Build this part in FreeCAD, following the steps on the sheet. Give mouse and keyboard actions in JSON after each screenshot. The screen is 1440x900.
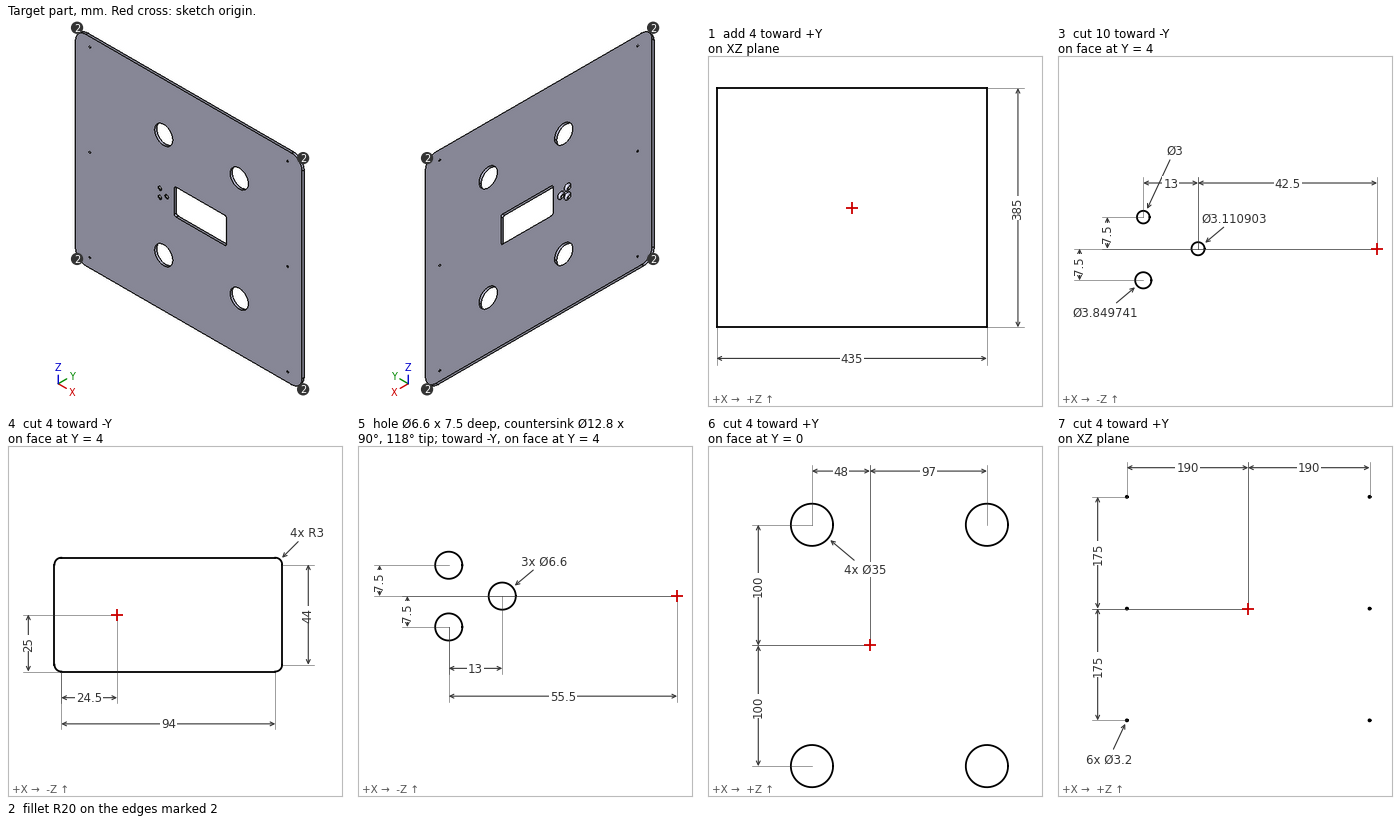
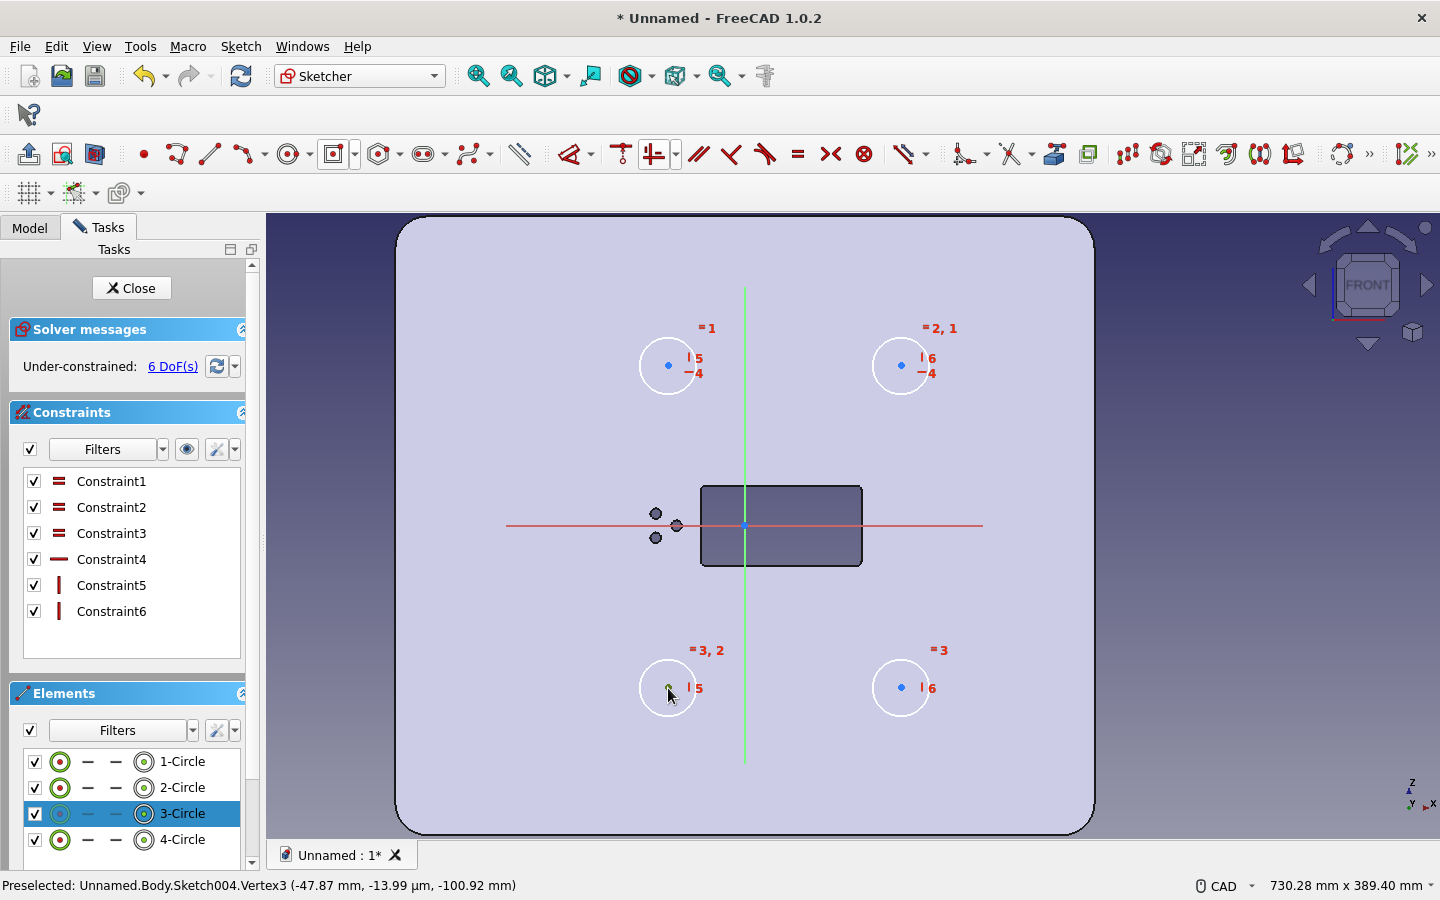
{"action": "left_click", "coordinate": [901, 688]}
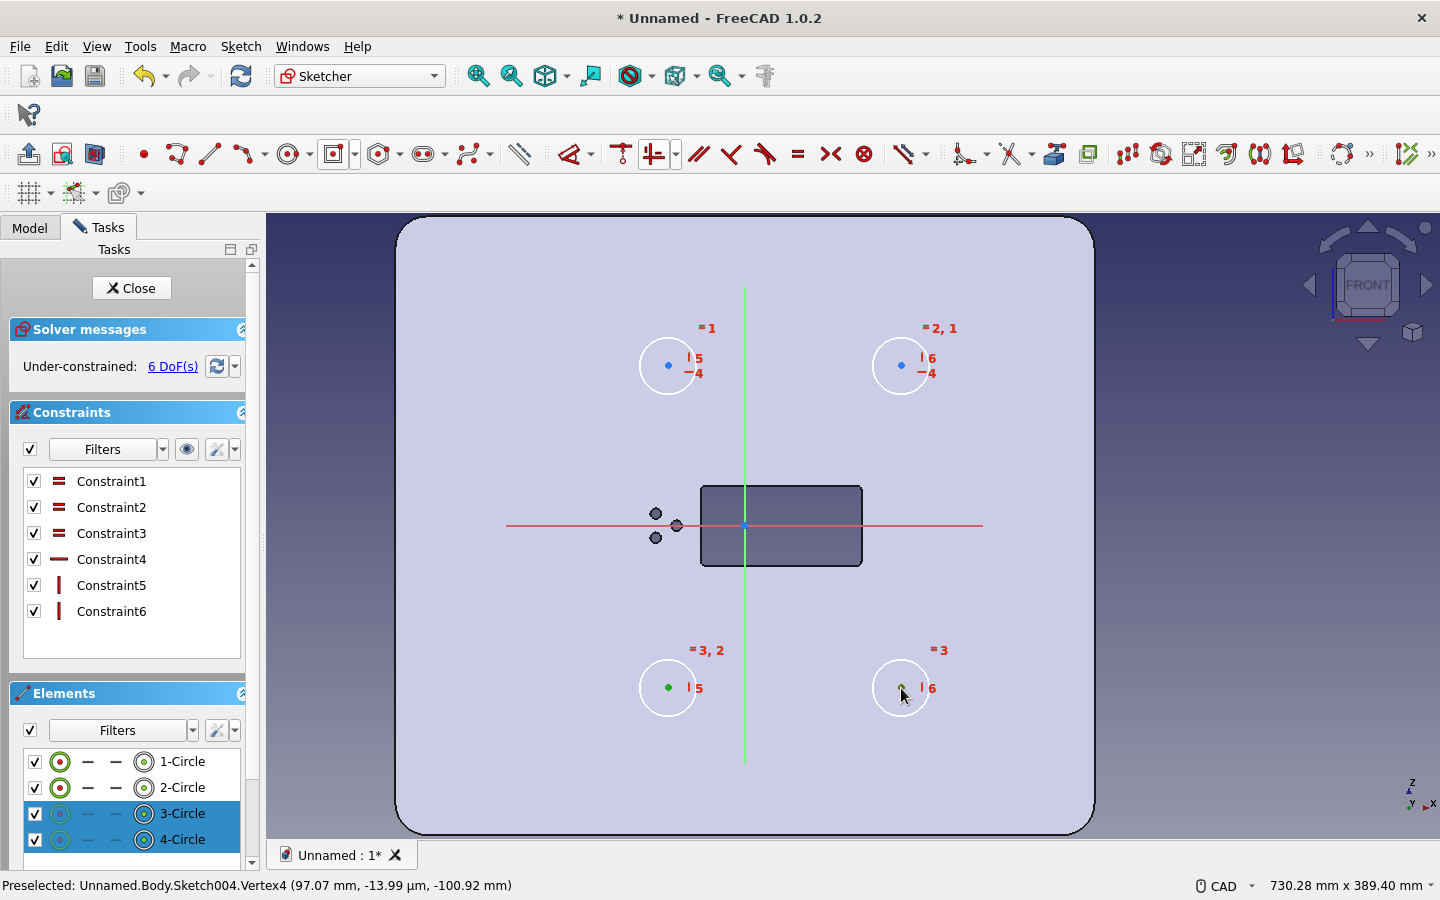
{"action": "left_click", "coordinate": [676, 154]}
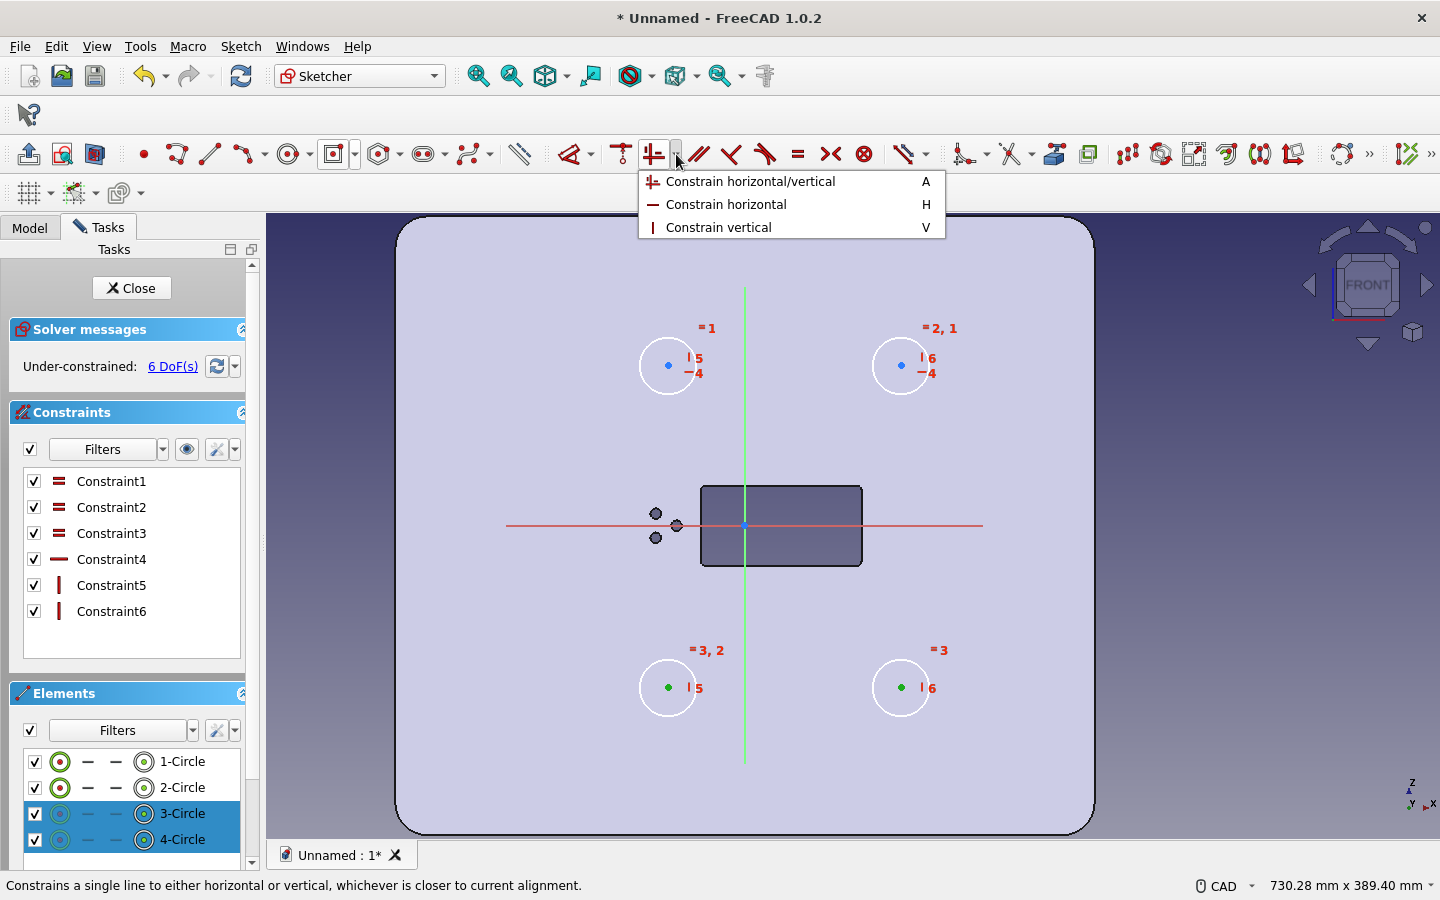
{"action": "left_click", "coordinate": [792, 204]}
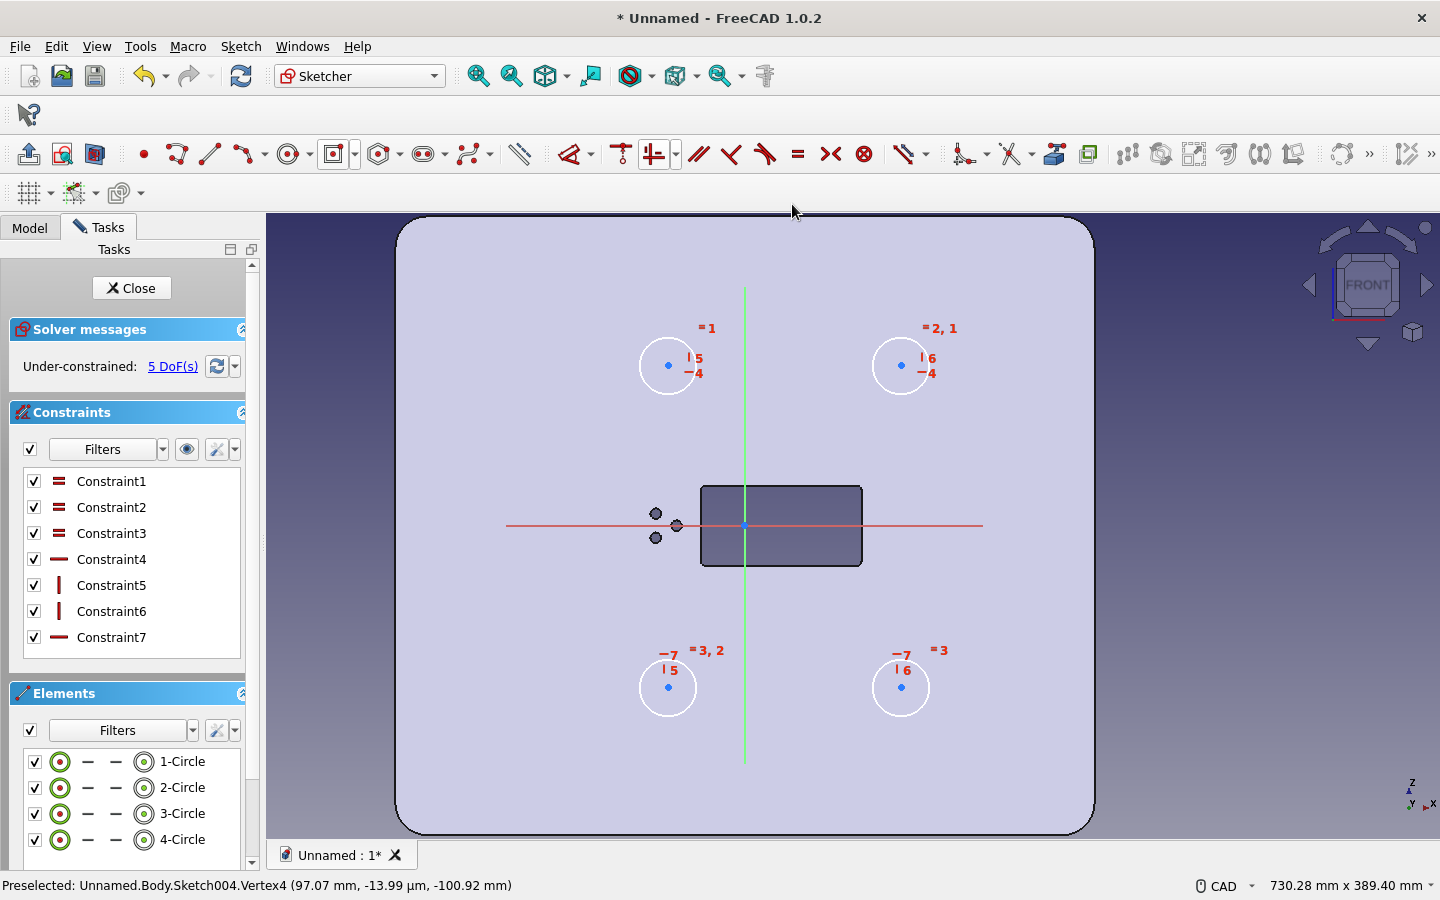
{"action": "left_click", "coordinate": [568, 154]}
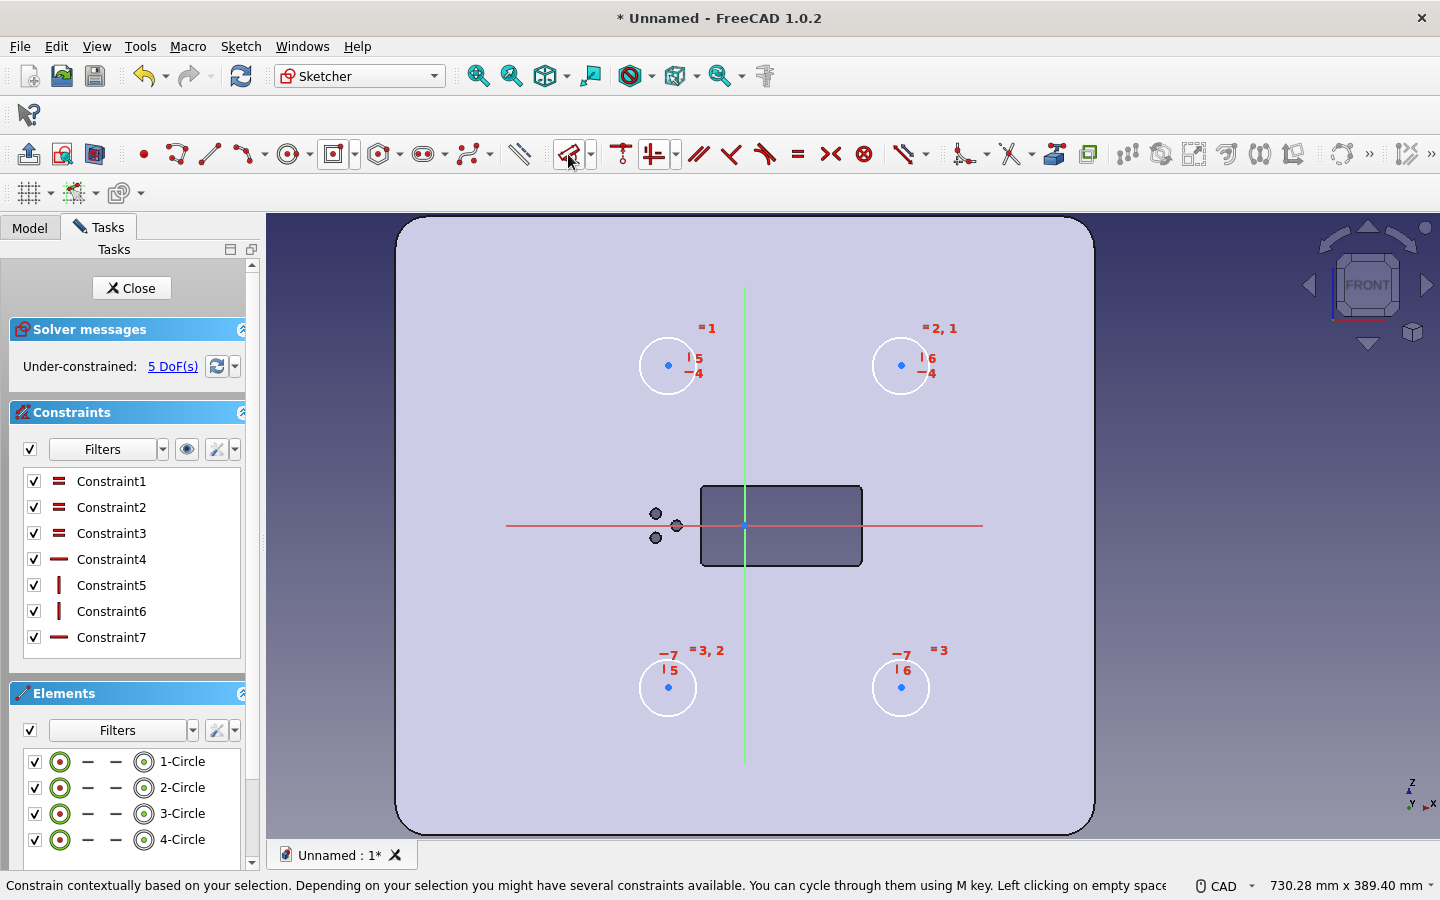
{"action": "left_click", "coordinate": [688, 346]}
{"action": "left_click", "coordinate": [711, 323]}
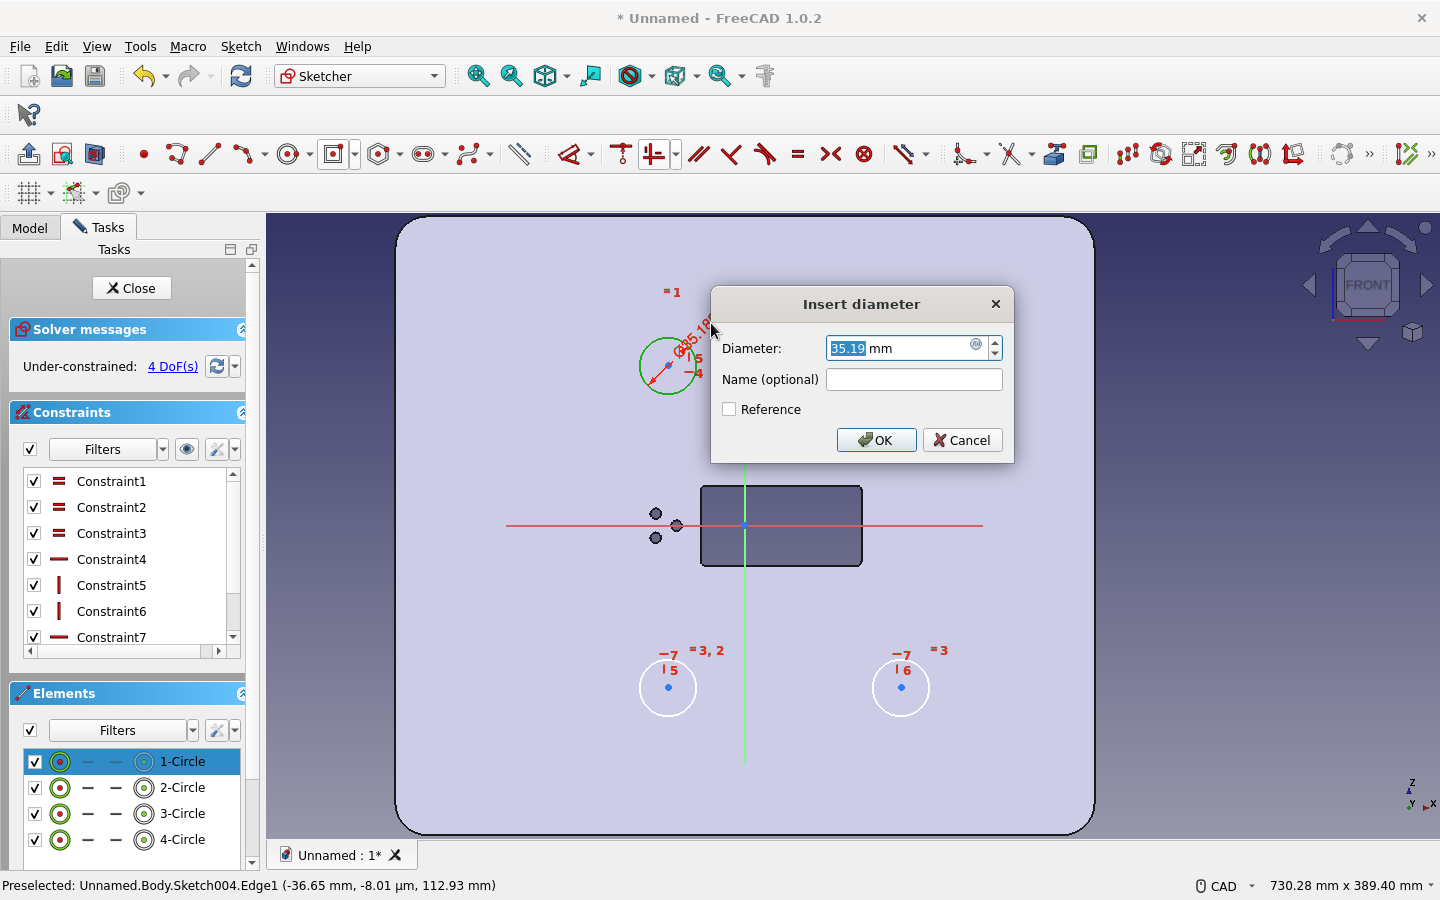
{"action": "type", "text": "35"}
{"action": "key", "text": "Return"}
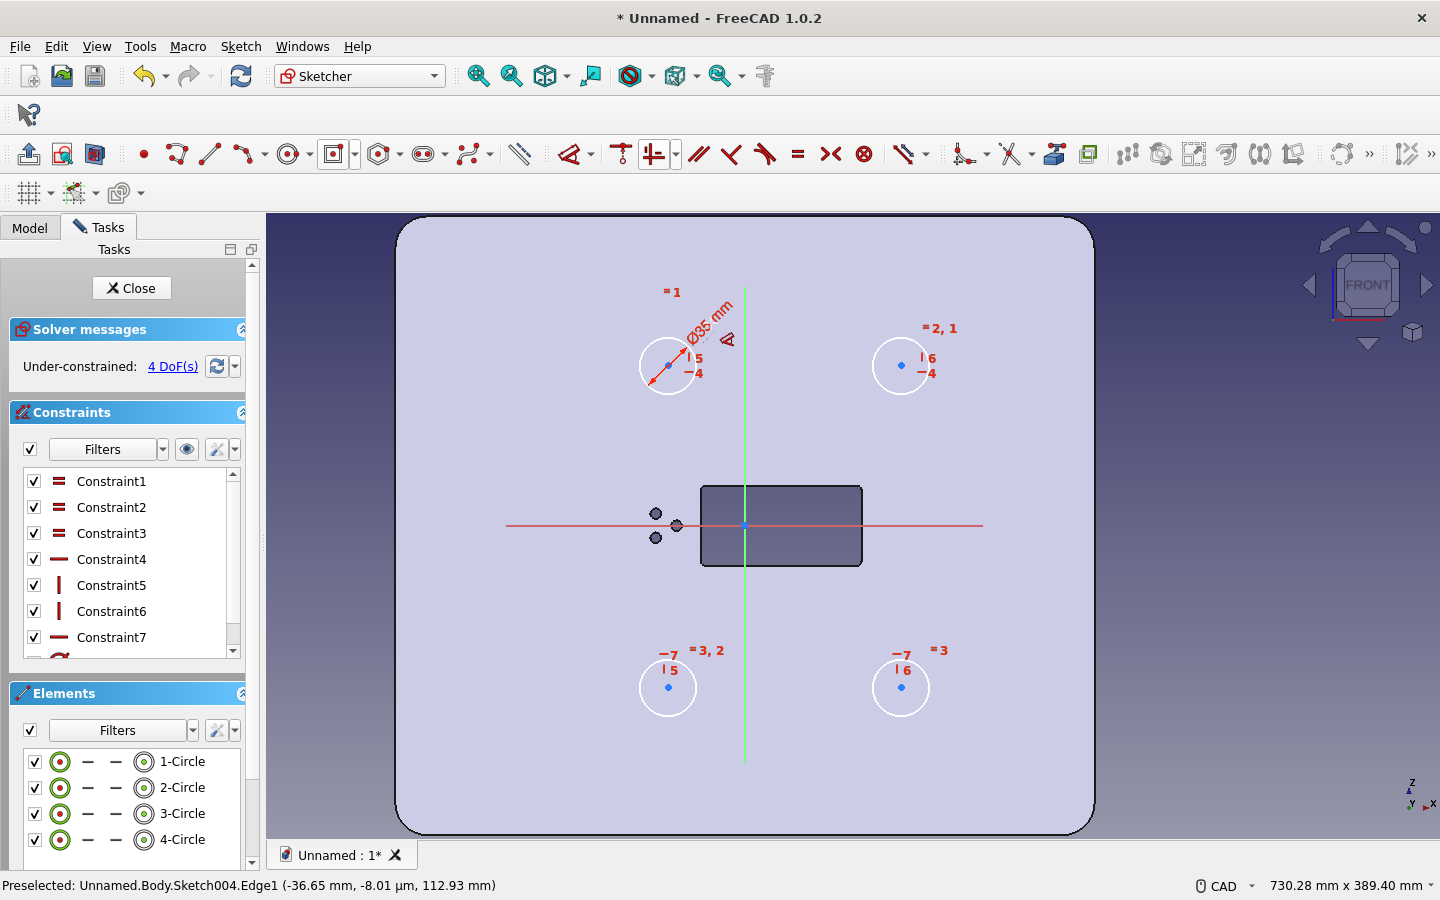
{"action": "left_click", "coordinate": [668, 366]}
{"action": "left_click", "coordinate": [706, 560]}